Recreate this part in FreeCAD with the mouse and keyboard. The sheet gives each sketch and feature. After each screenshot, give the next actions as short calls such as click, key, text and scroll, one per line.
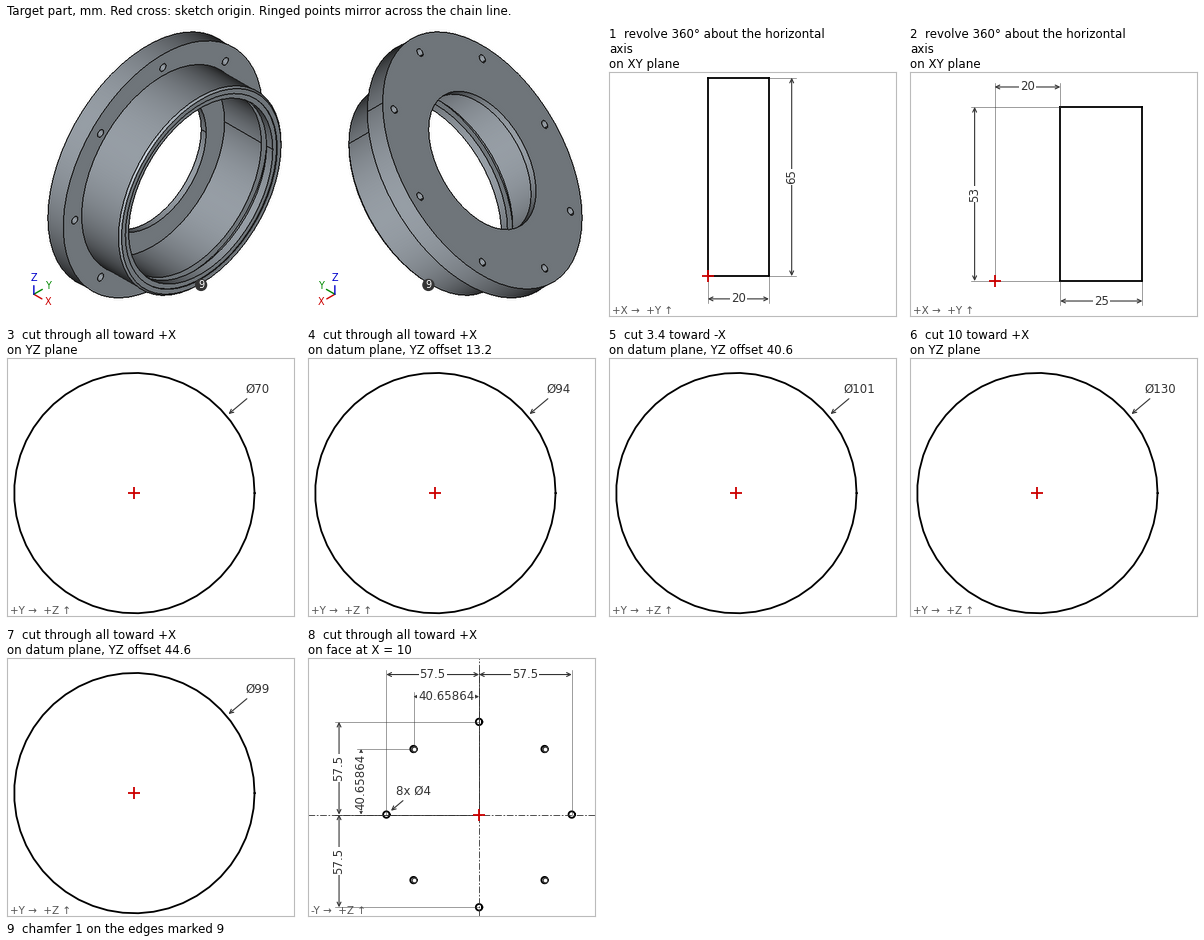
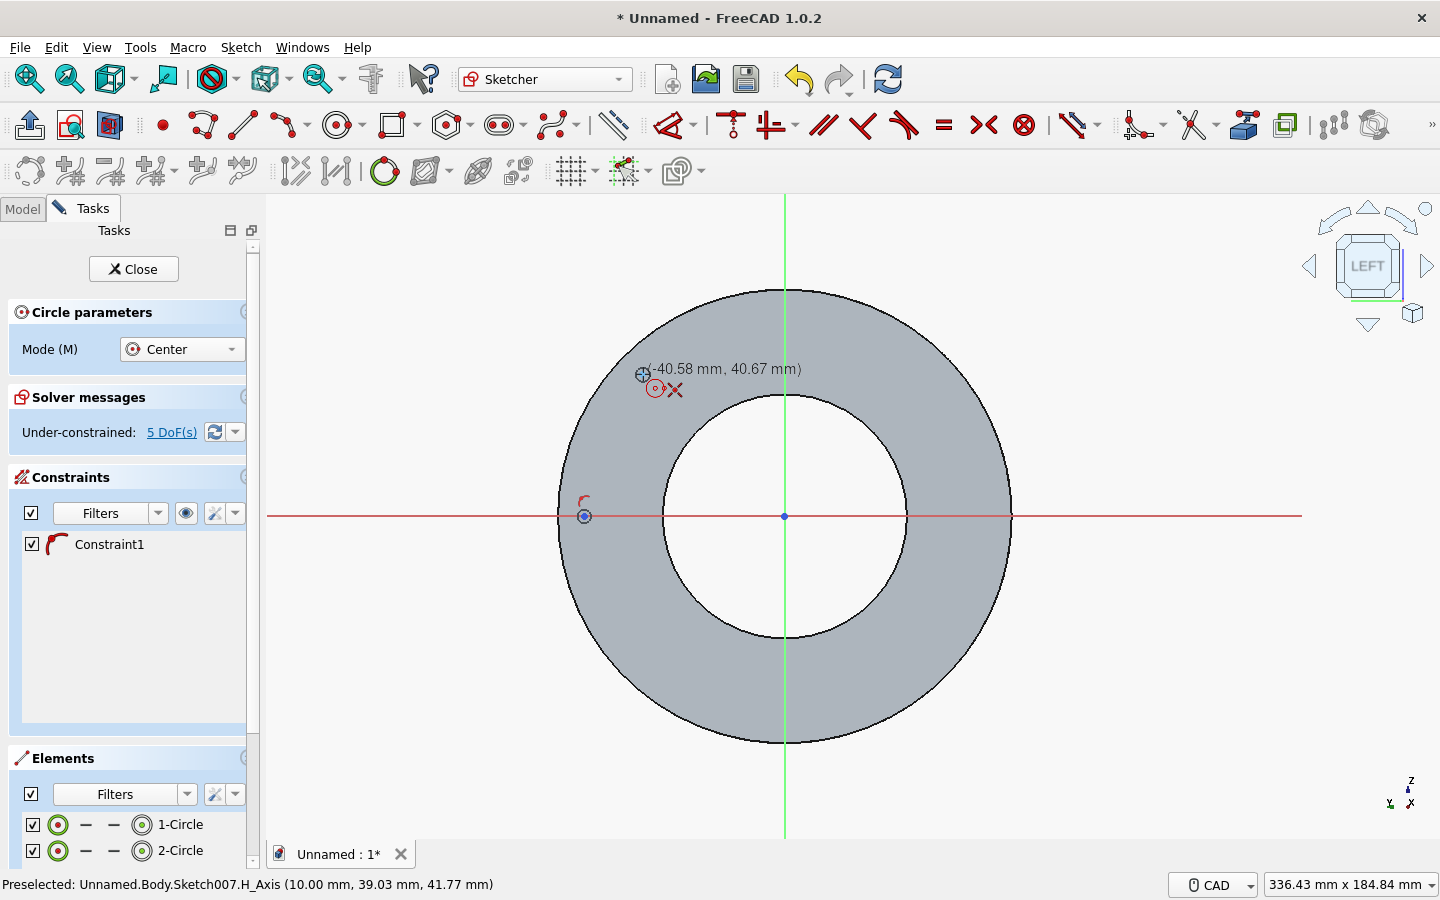
scroll(785, 316, up, 6)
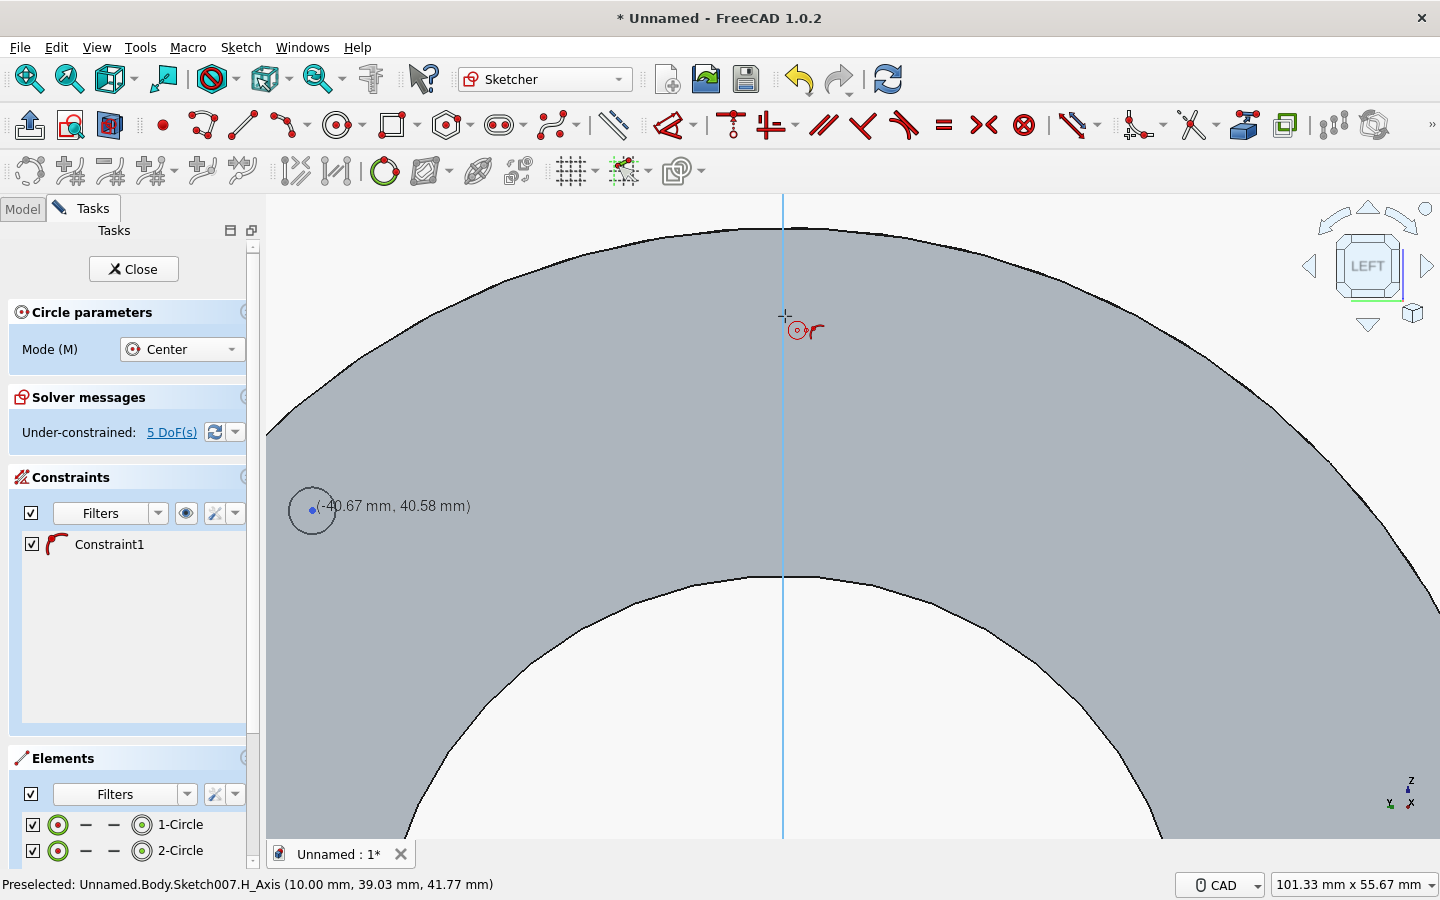
click(783, 315)
click(800, 298)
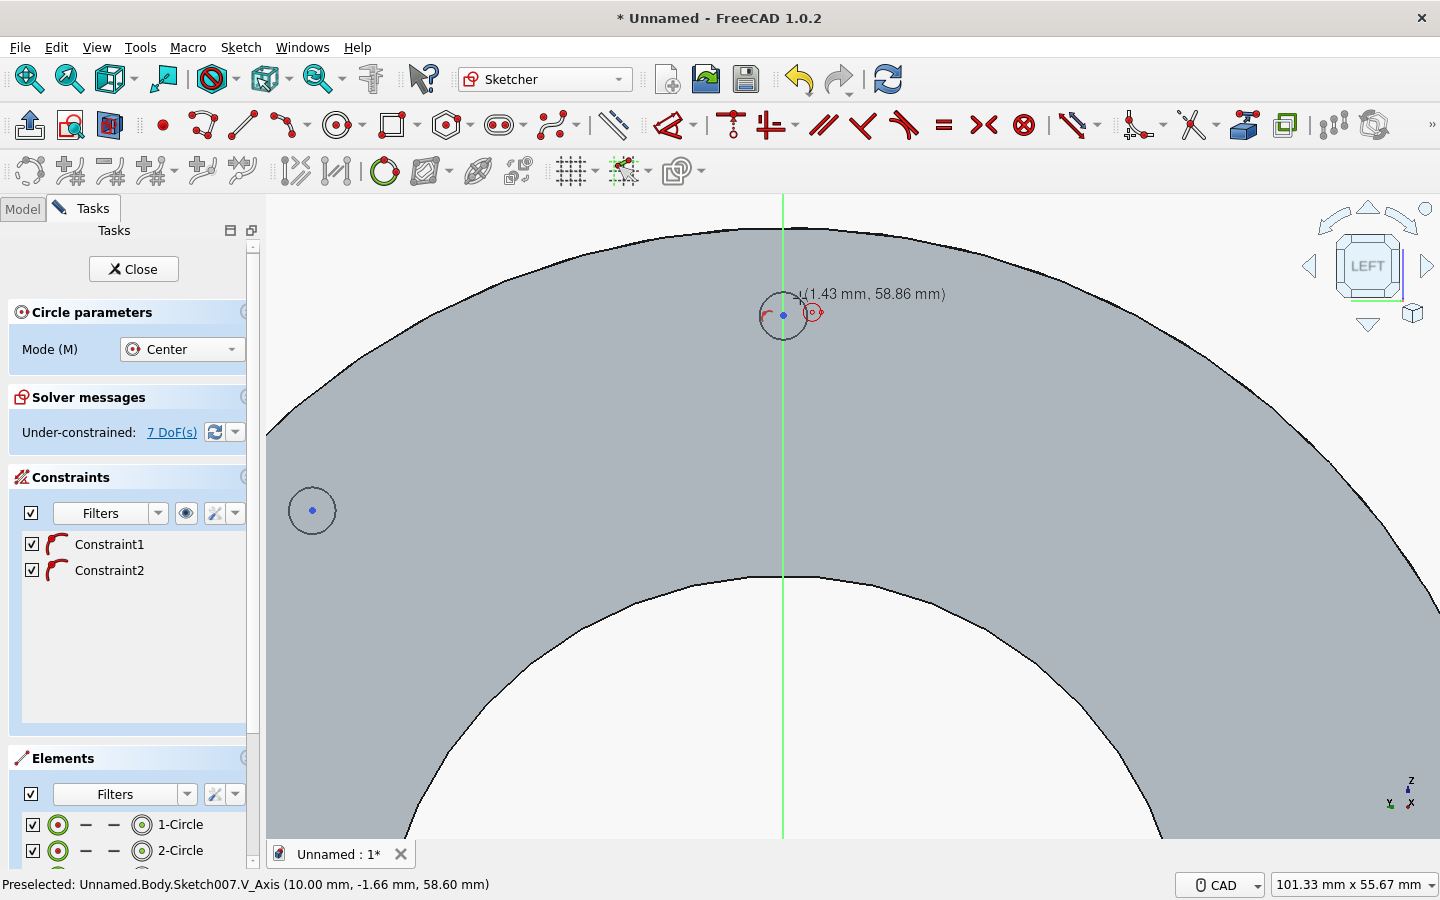
click(1255, 510)
click(1271, 494)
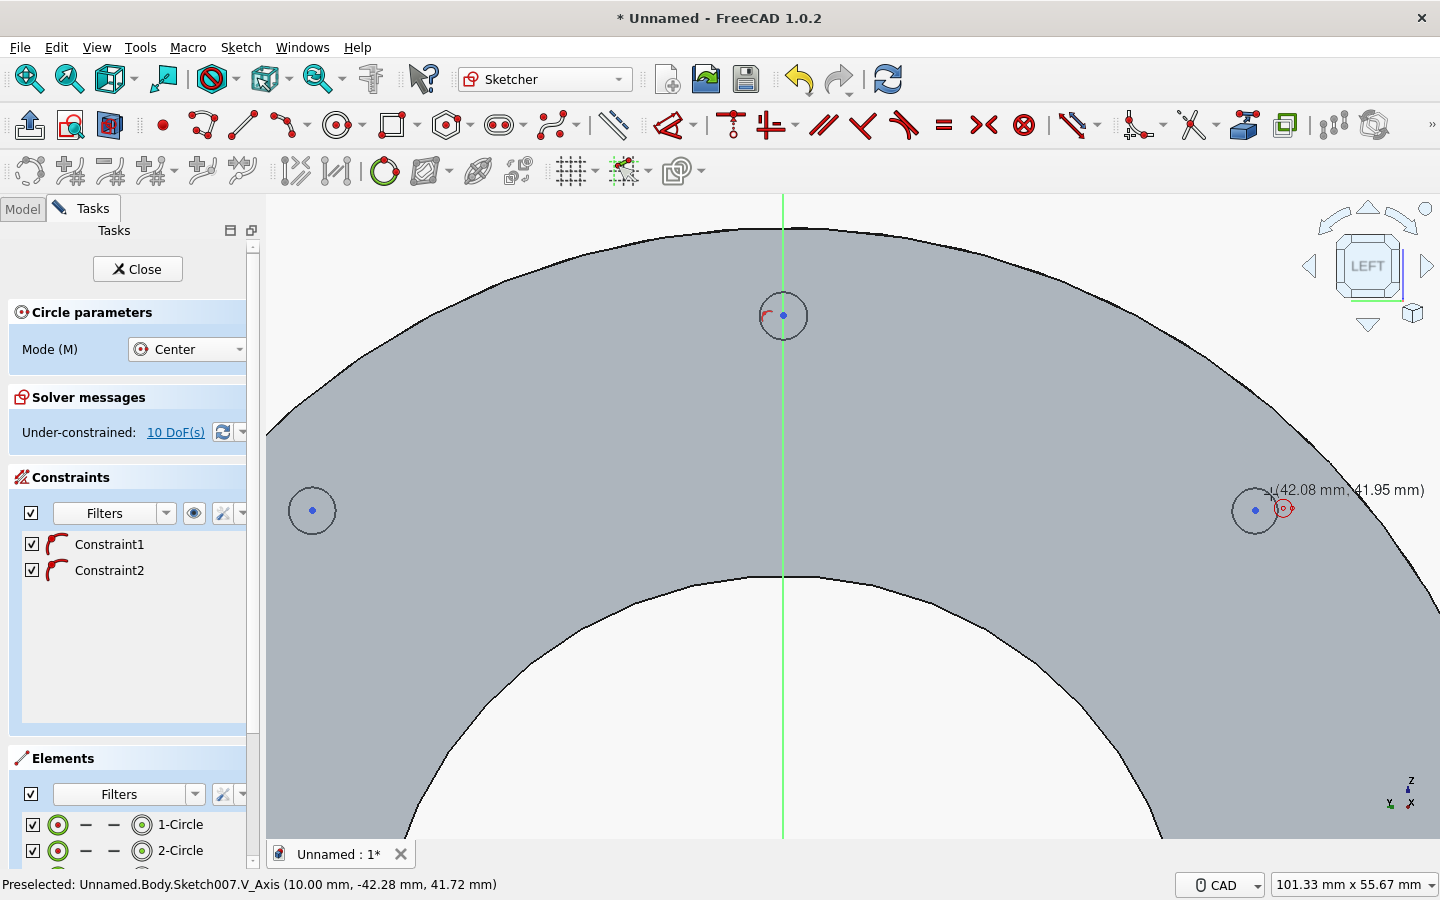
scroll(785, 316, down, 6)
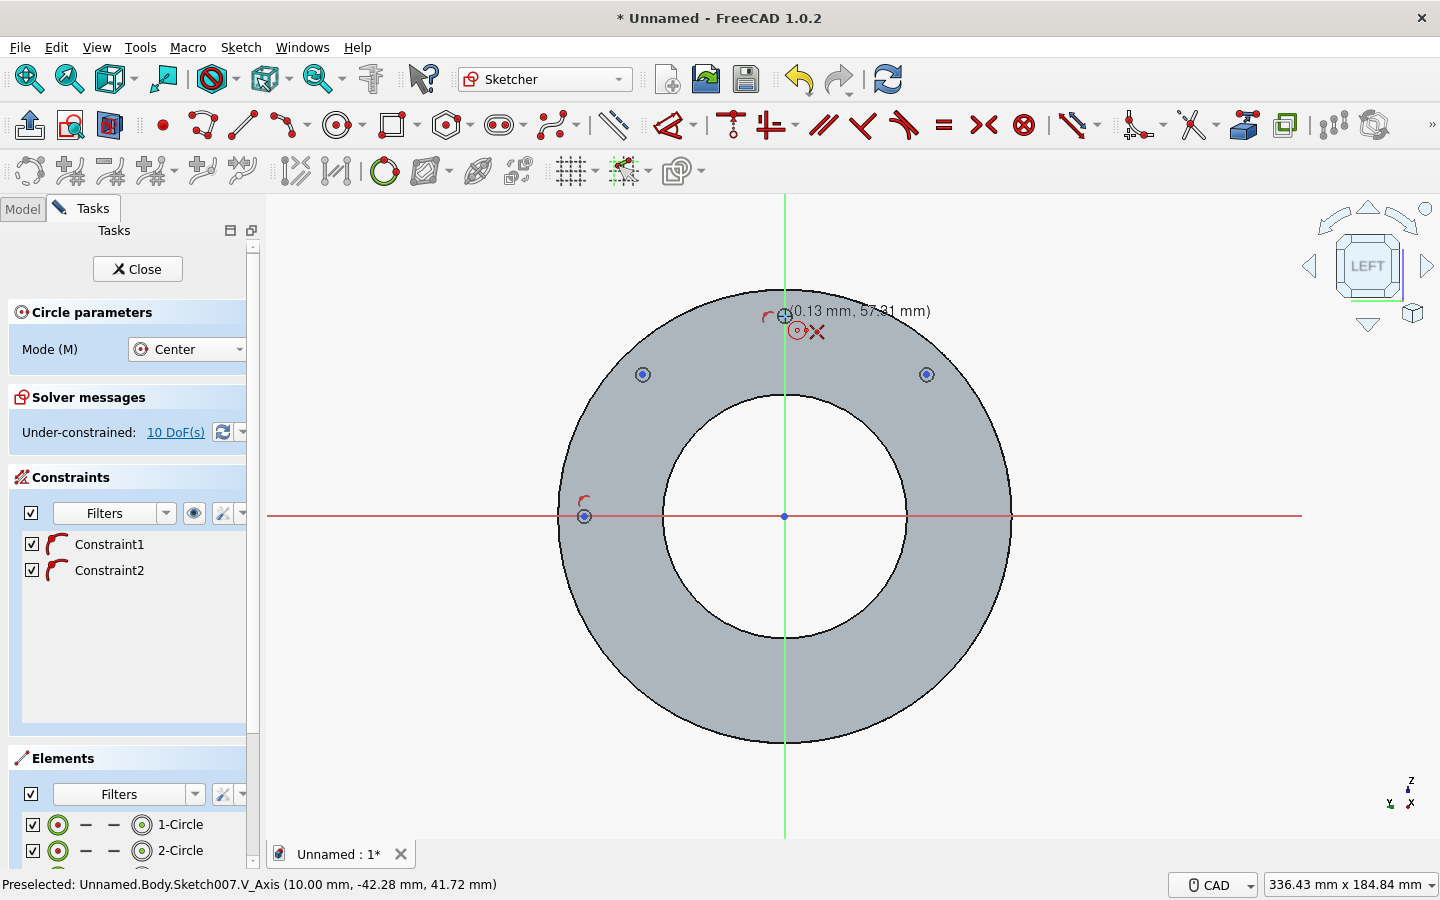
scroll(985, 516, up, 6)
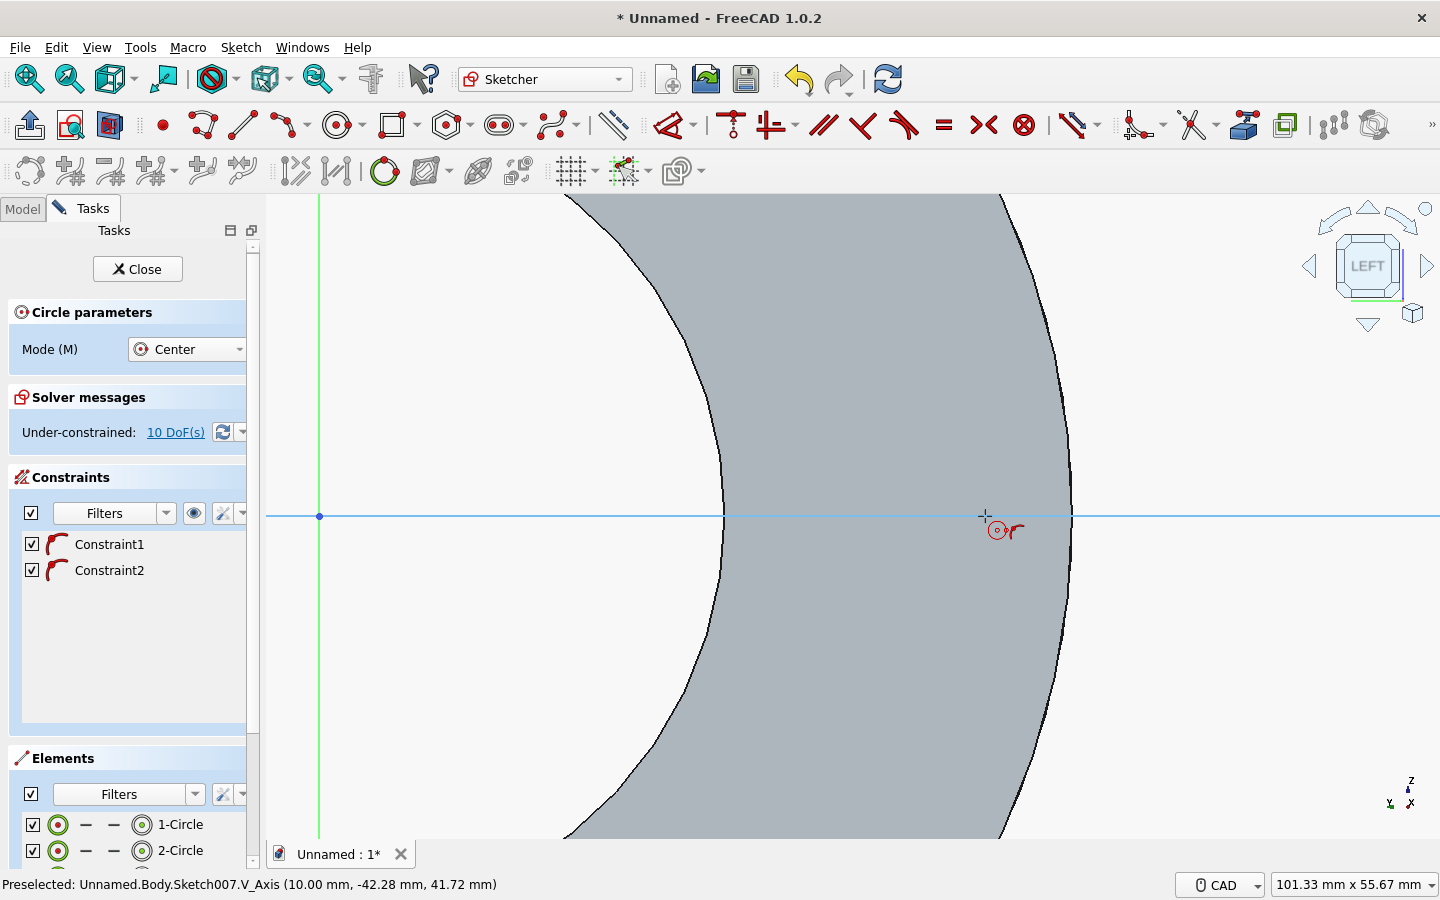
click(985, 516)
click(1002, 500)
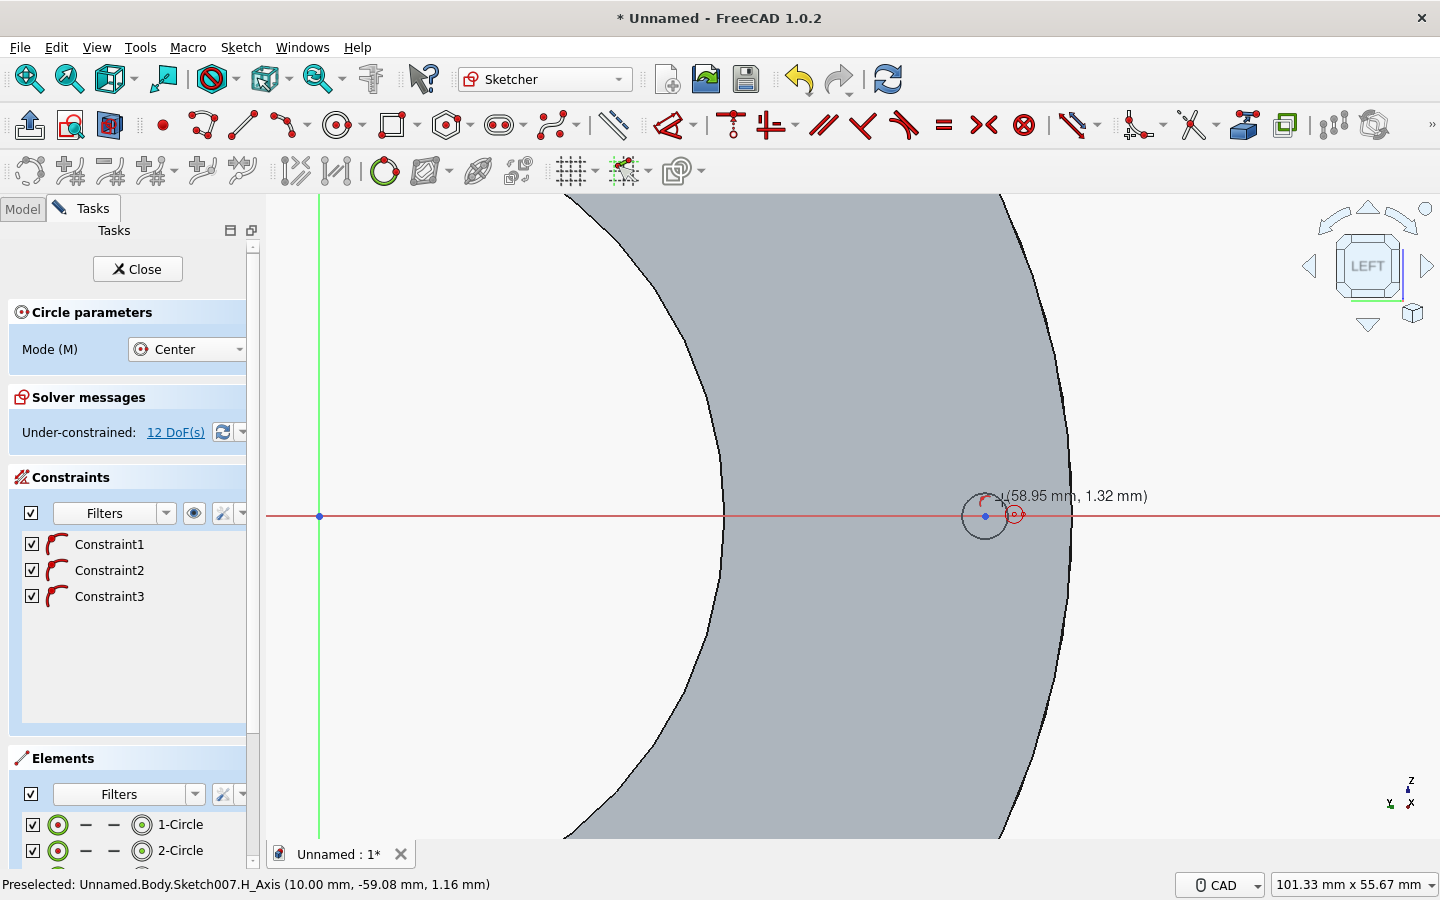
scroll(985, 517, down, 6)